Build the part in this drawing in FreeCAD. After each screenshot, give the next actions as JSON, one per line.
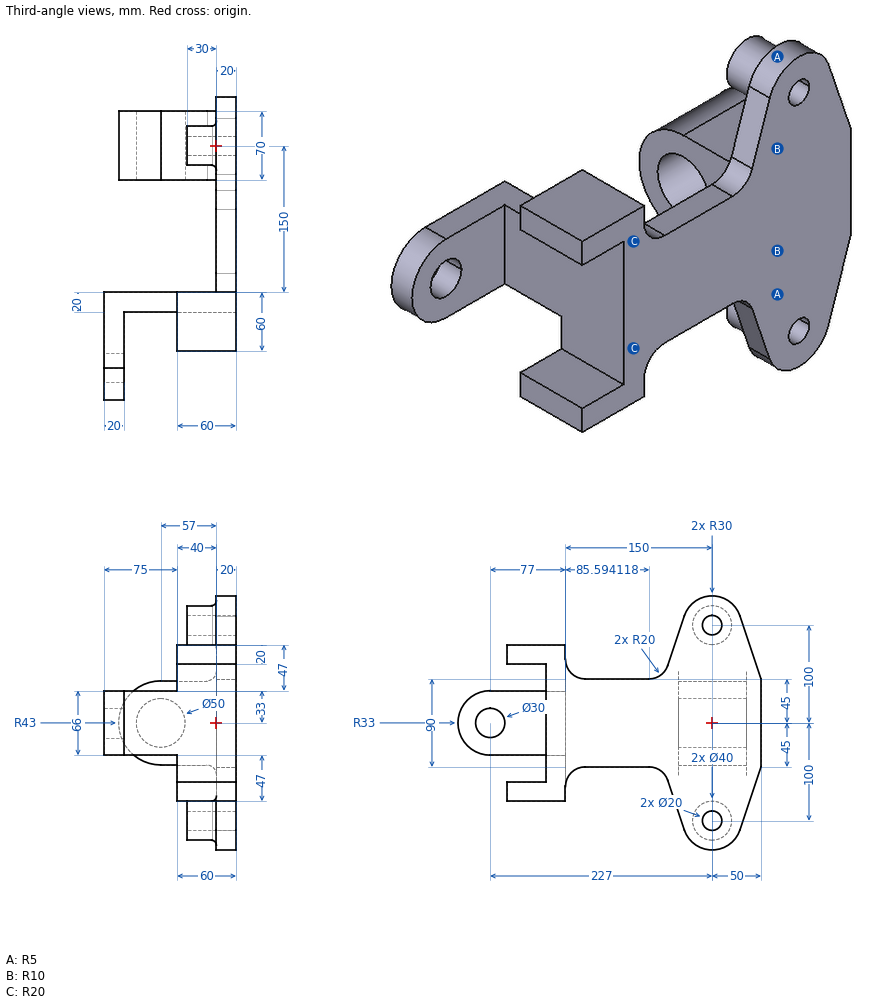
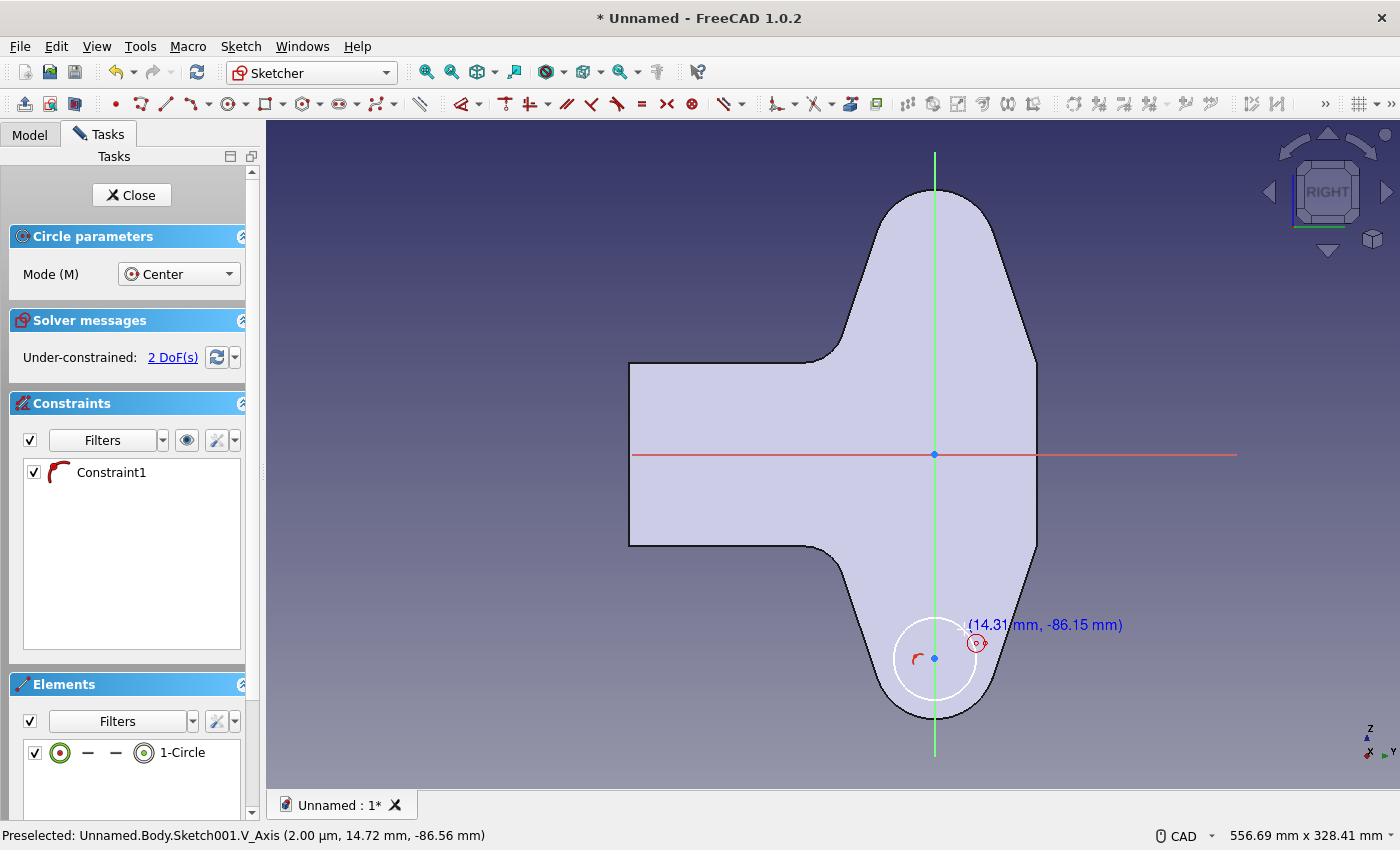
{"action": "left_click", "coordinate": [935, 251]}
{"action": "left_click", "coordinate": [964, 222]}
{"action": "key", "text": "Escape"}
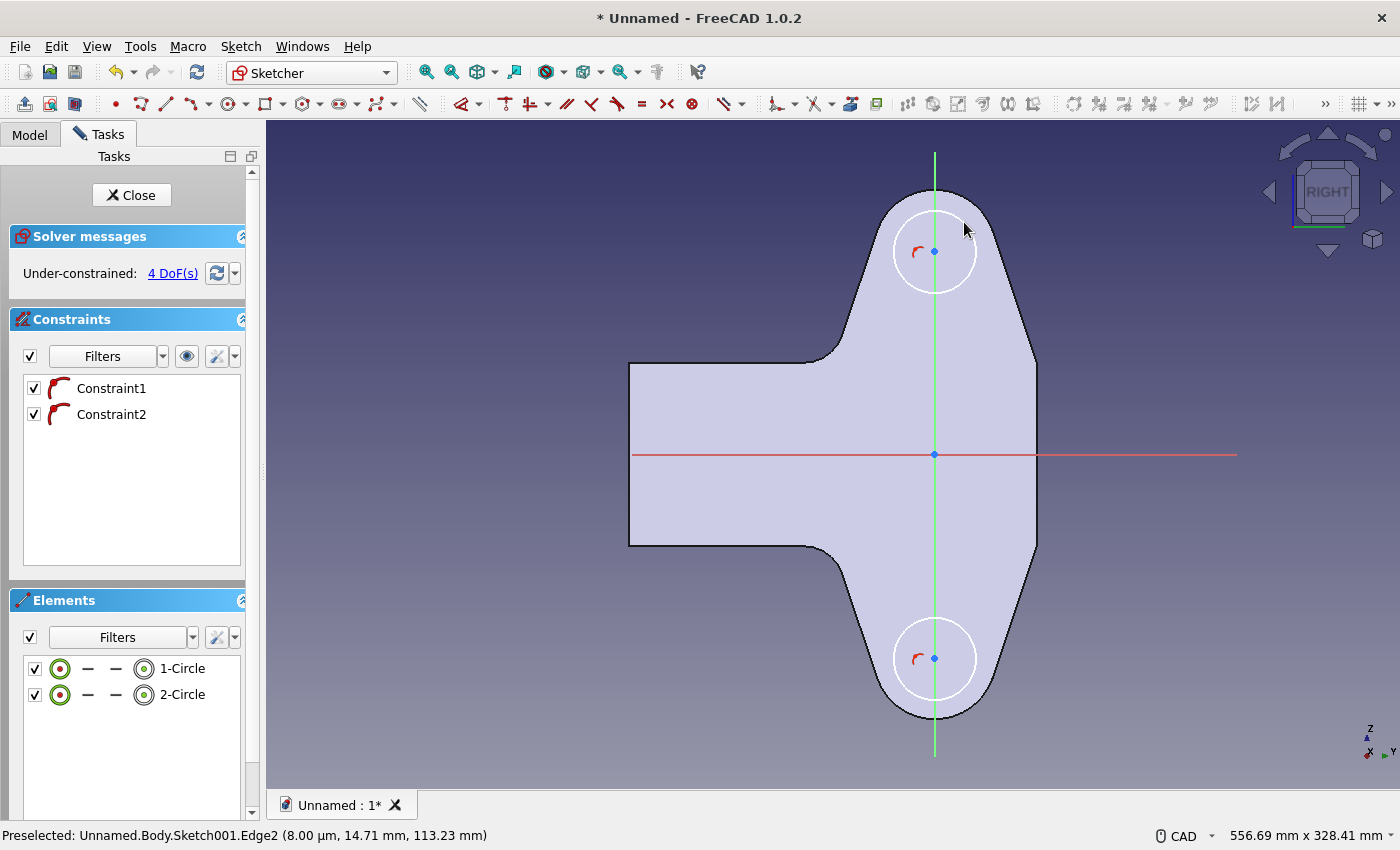
{"action": "left_click", "coordinate": [964, 630]}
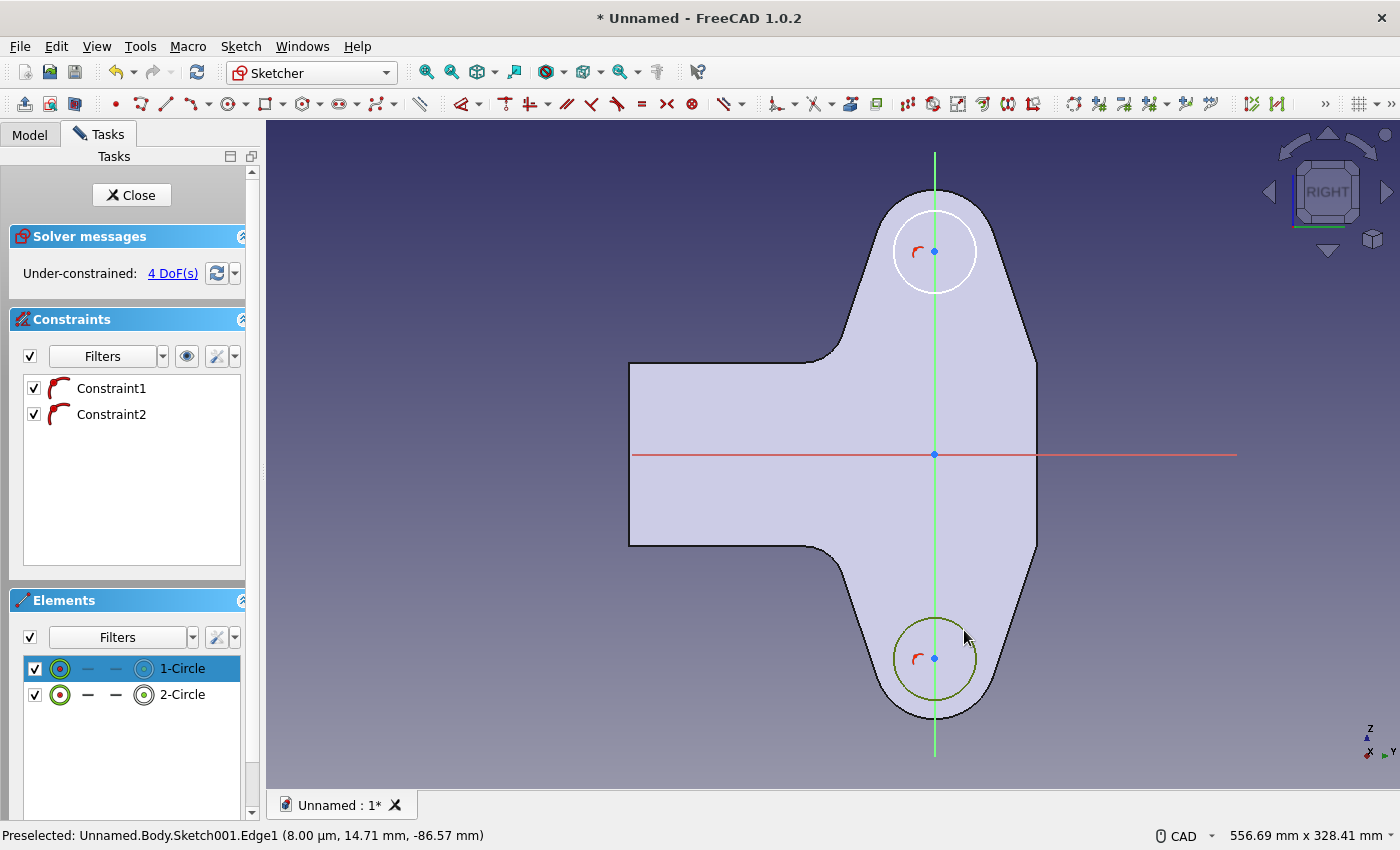
{"action": "left_click", "coordinate": [964, 223]}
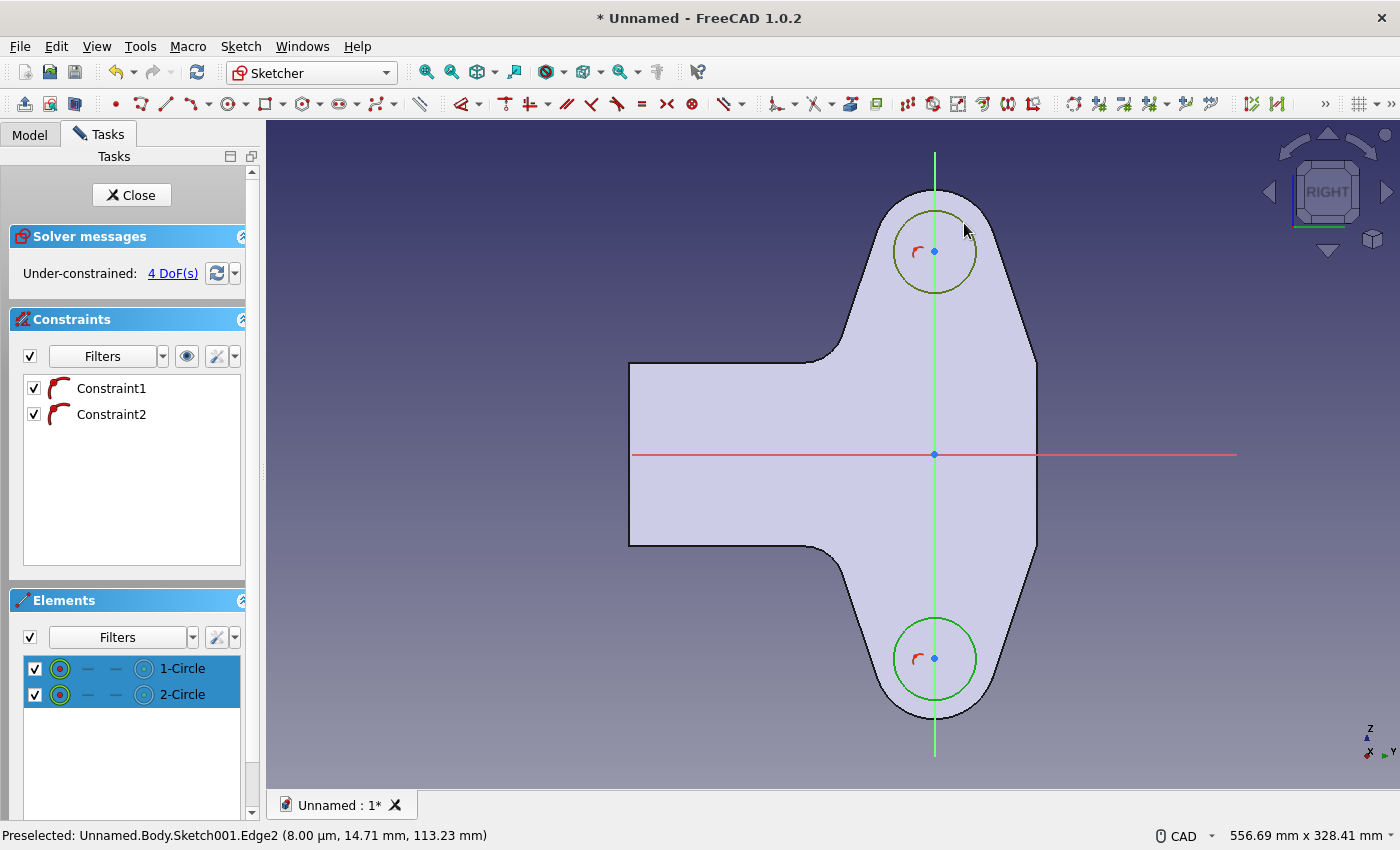
{"action": "key", "text": "e"}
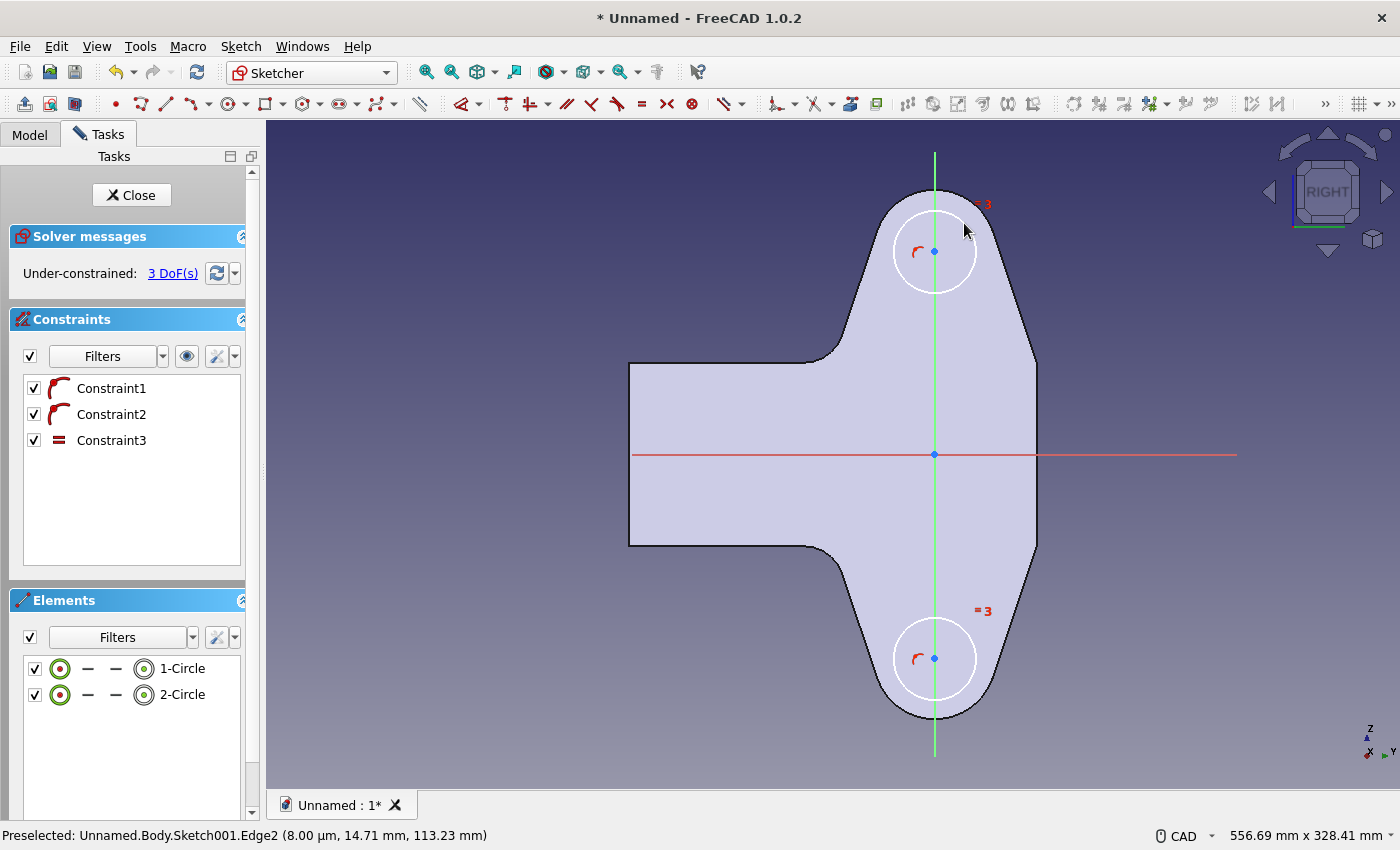
{"action": "left_click", "coordinate": [460, 104]}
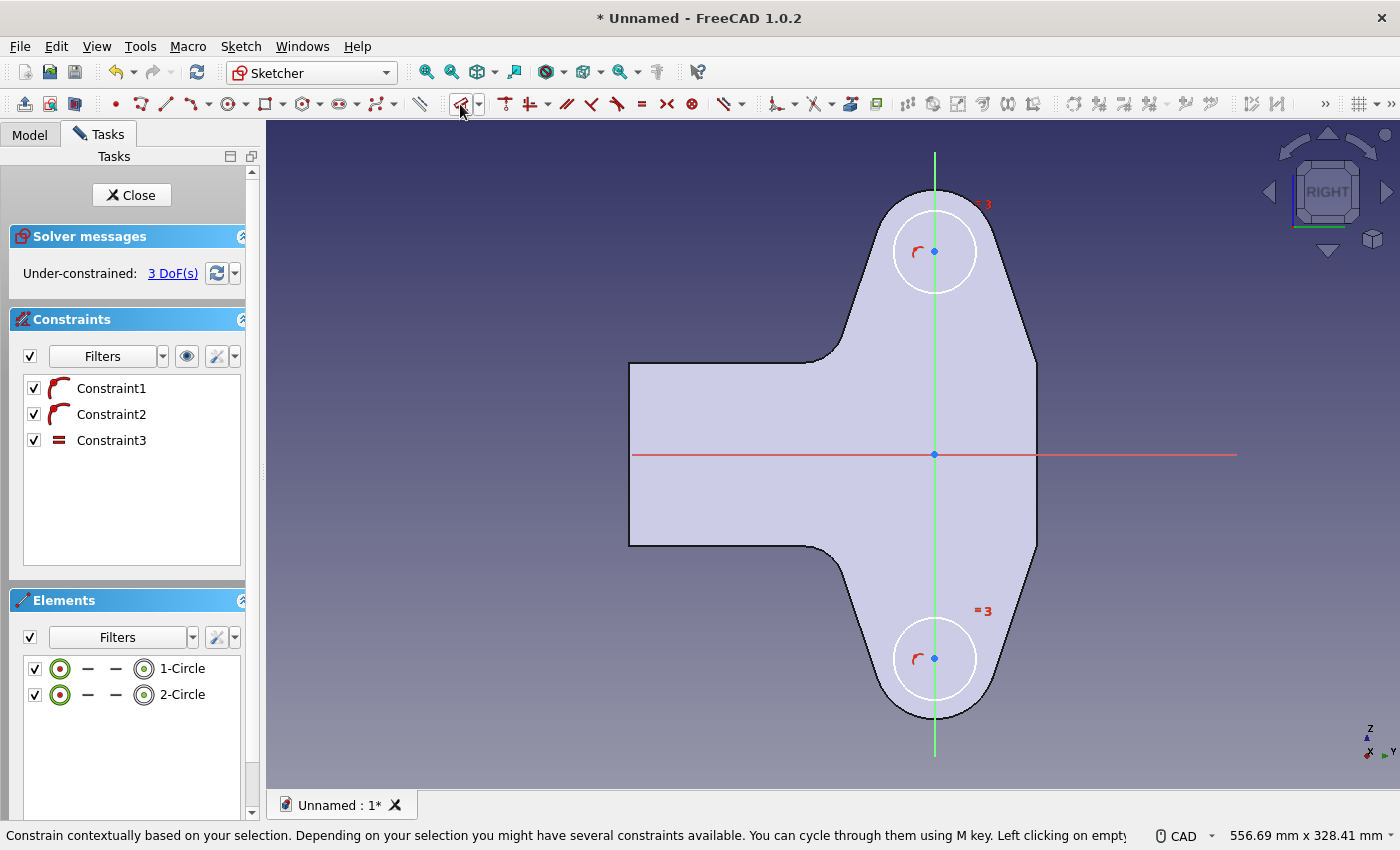
{"action": "left_click", "coordinate": [964, 630]}
{"action": "left_click", "coordinate": [987, 607]}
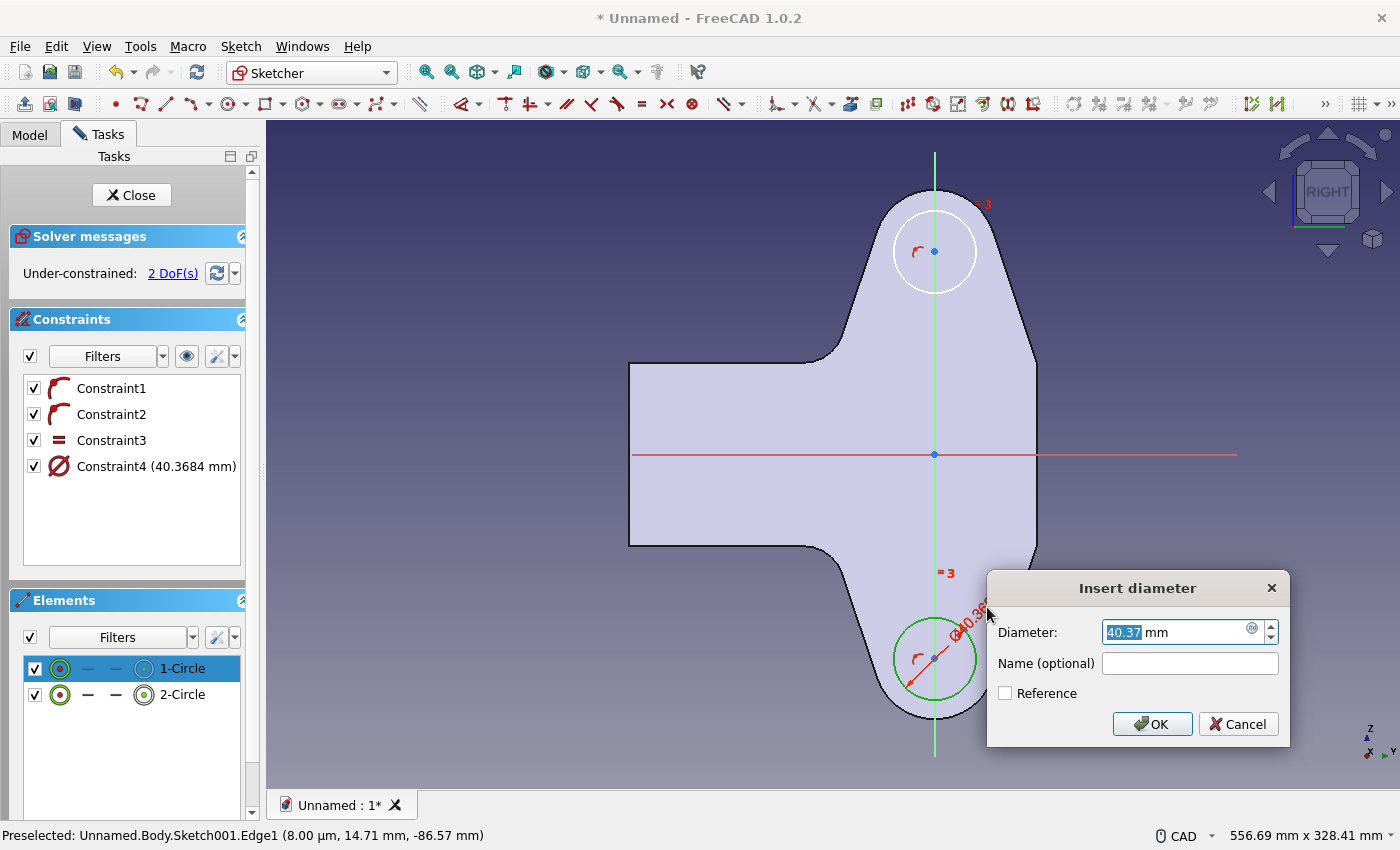
{"action": "type", "text": "40"}
{"action": "key", "text": "Return"}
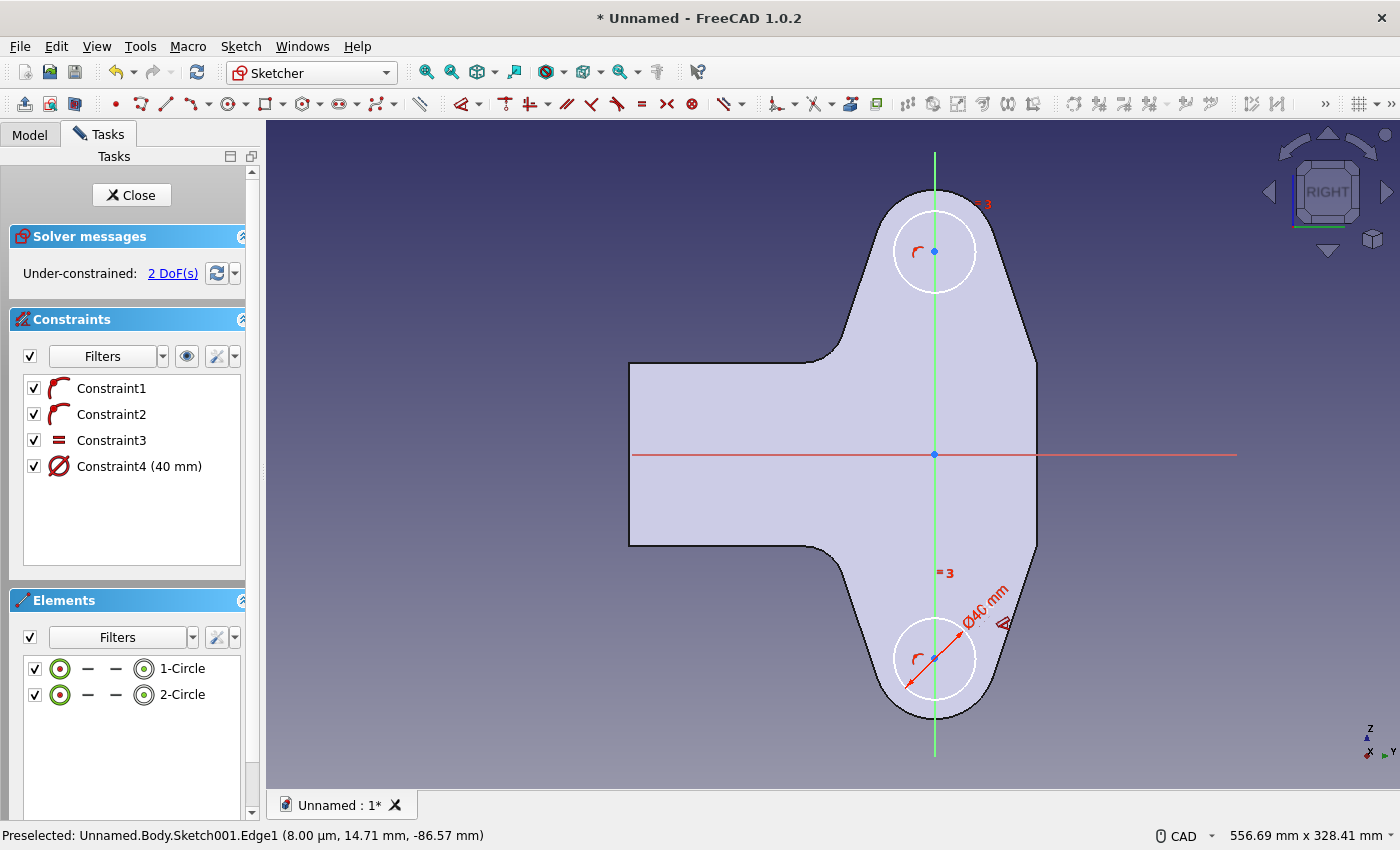
{"action": "left_click", "coordinate": [935, 659]}
{"action": "left_click", "coordinate": [969, 557]}